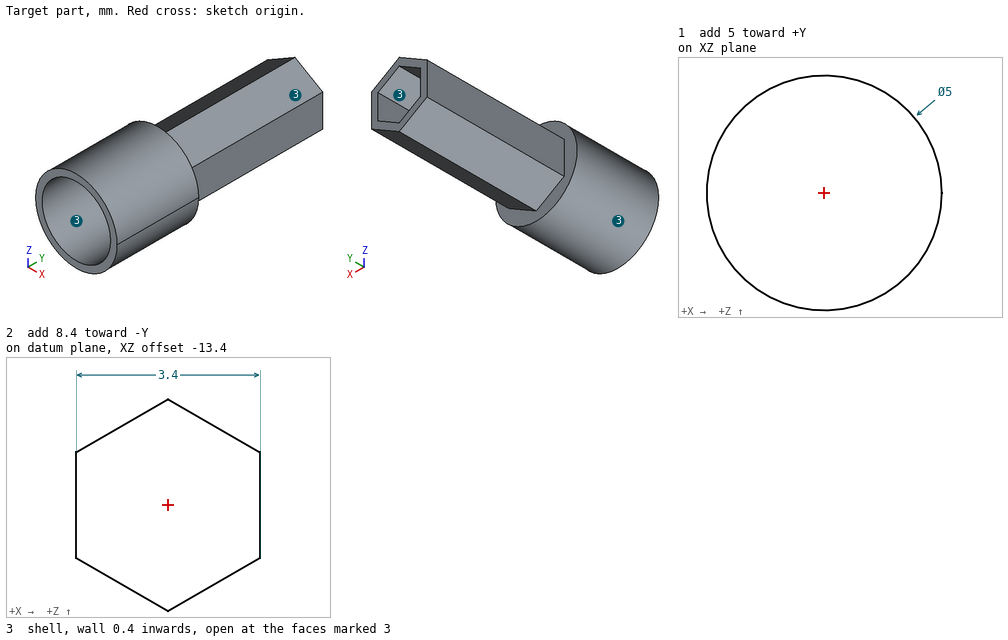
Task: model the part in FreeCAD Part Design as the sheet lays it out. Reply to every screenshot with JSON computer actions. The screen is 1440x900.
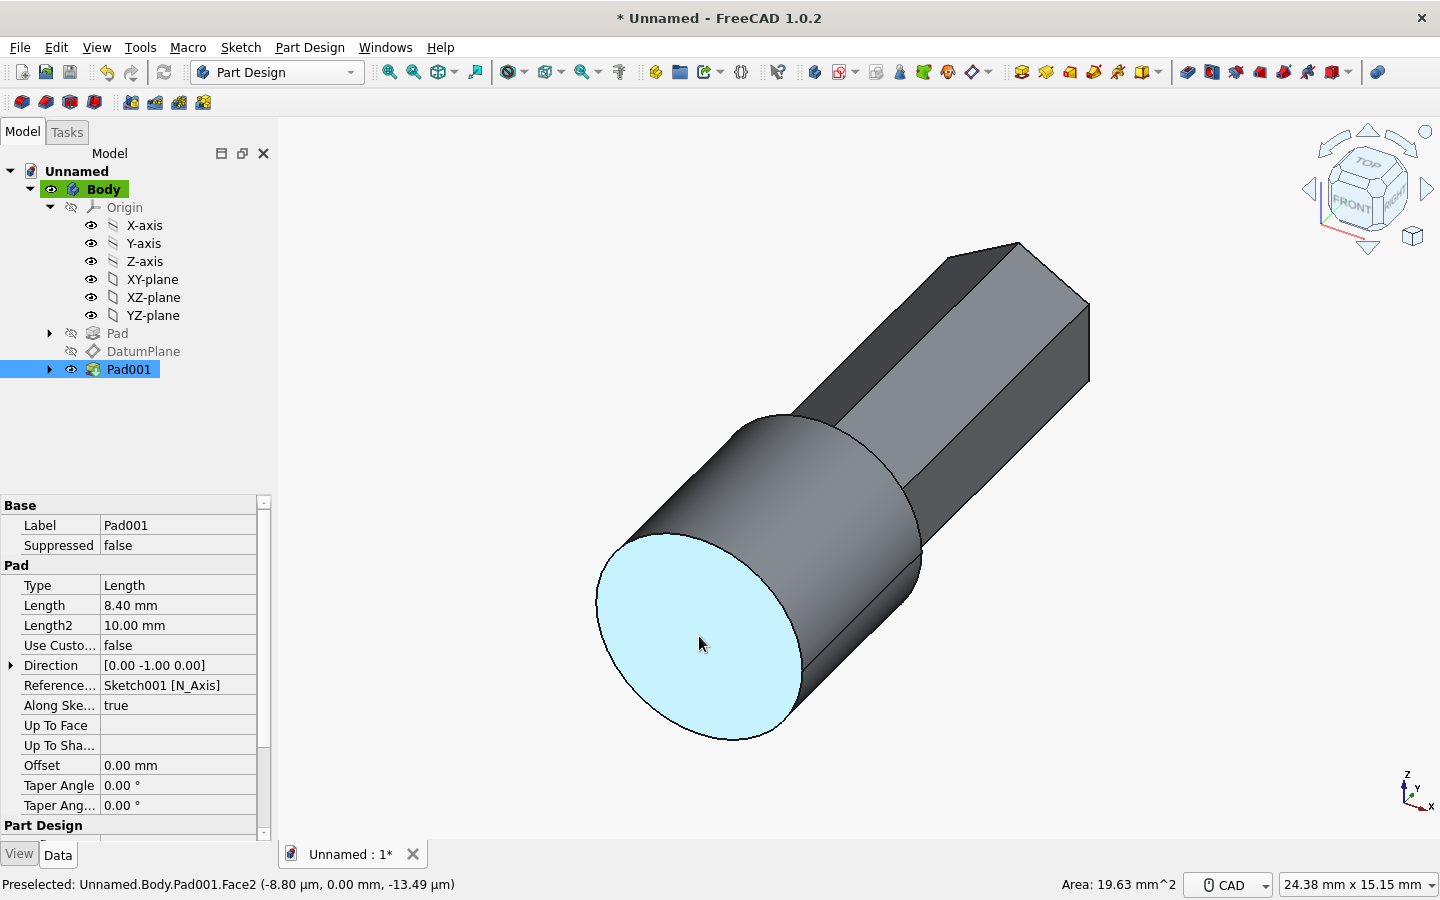
{"action": "key", "text": "0"}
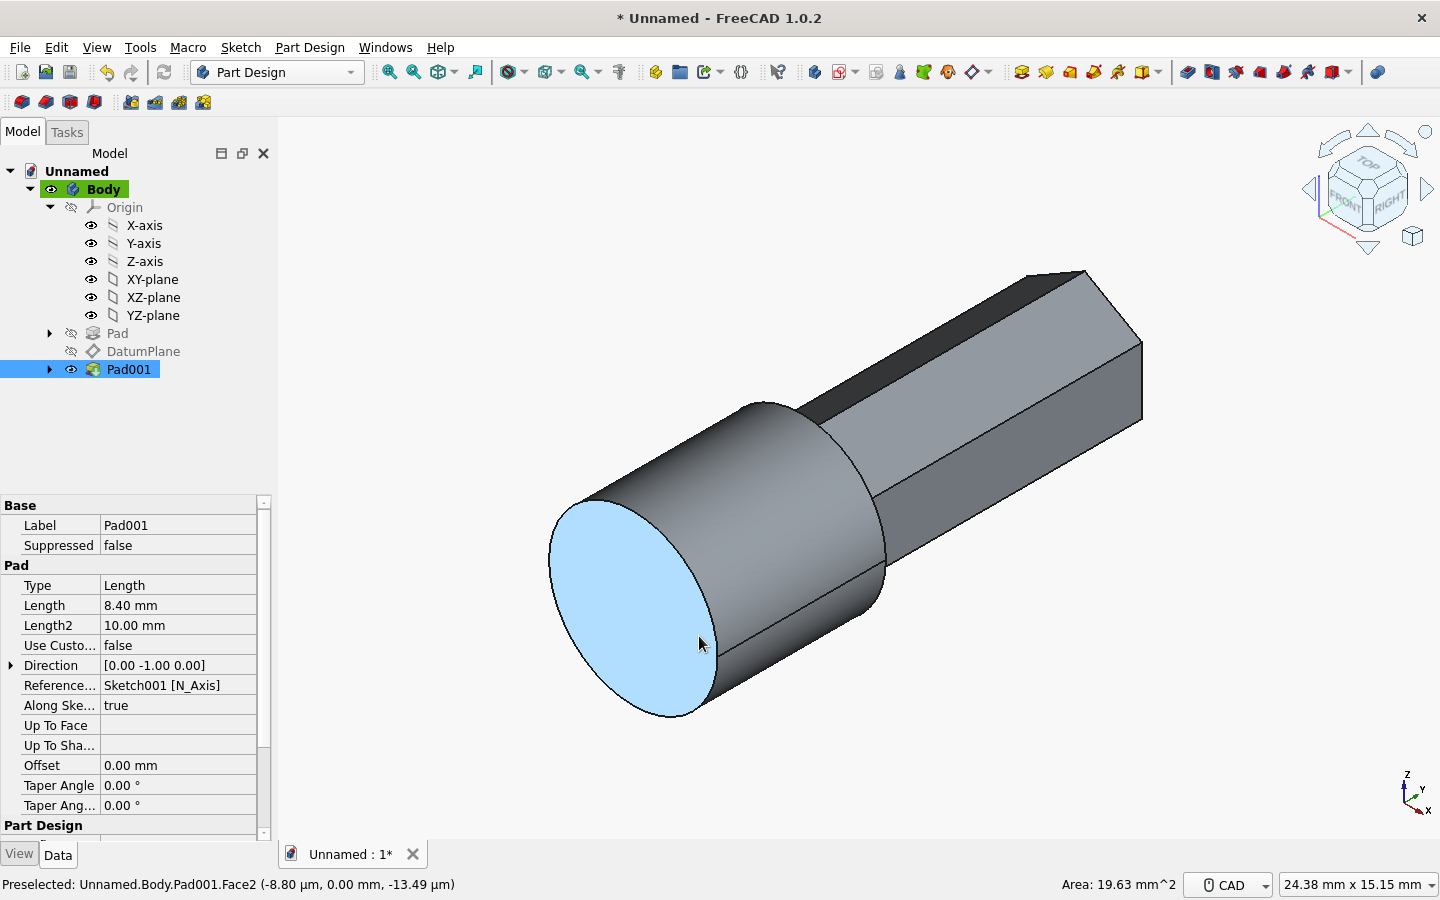
{"action": "key", "text": "2"}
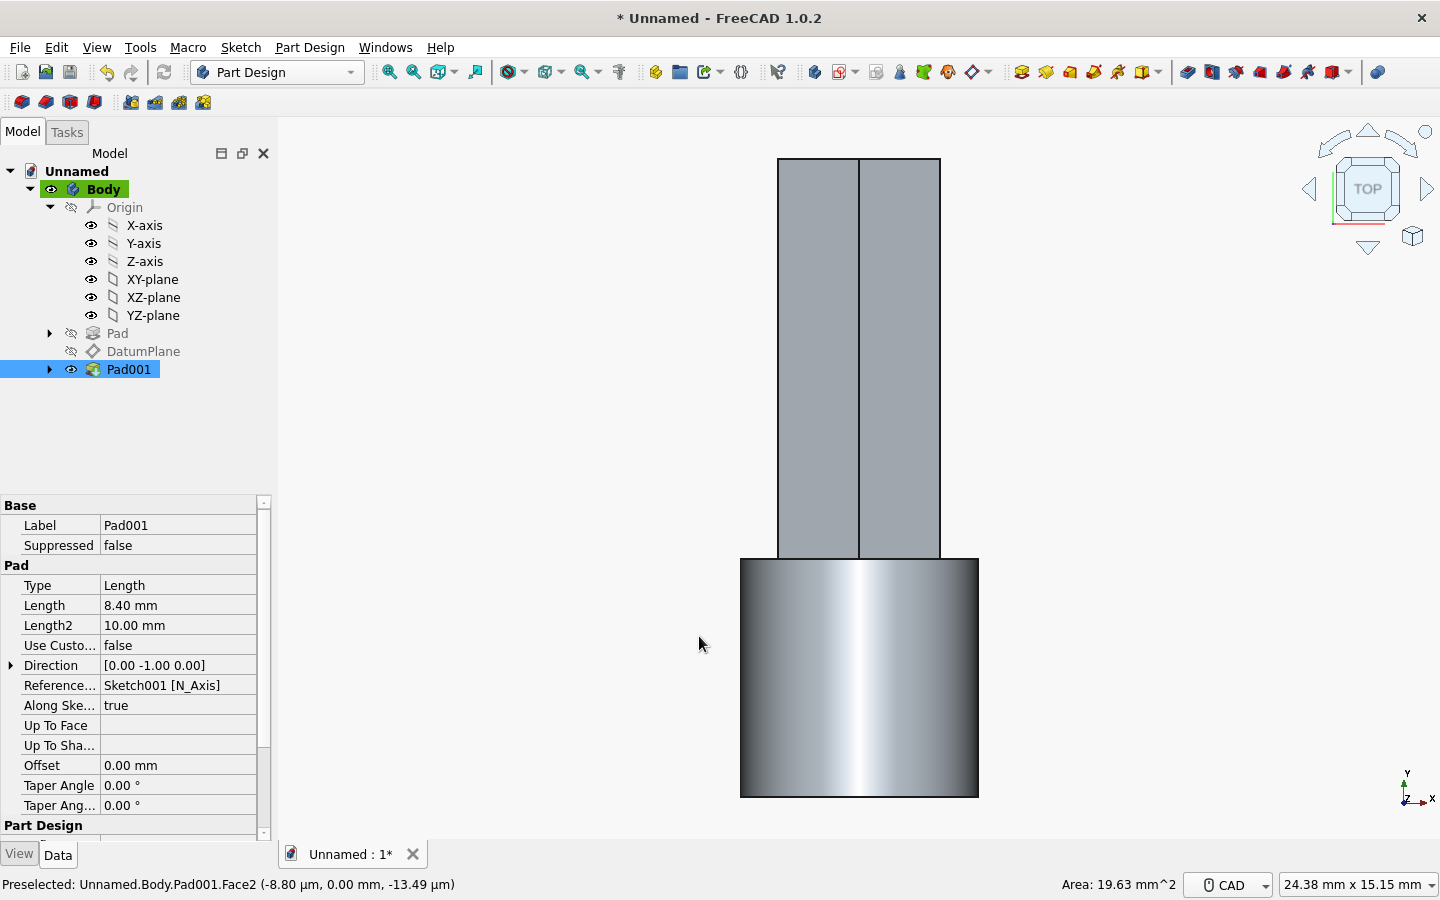
{"action": "key", "text": "1"}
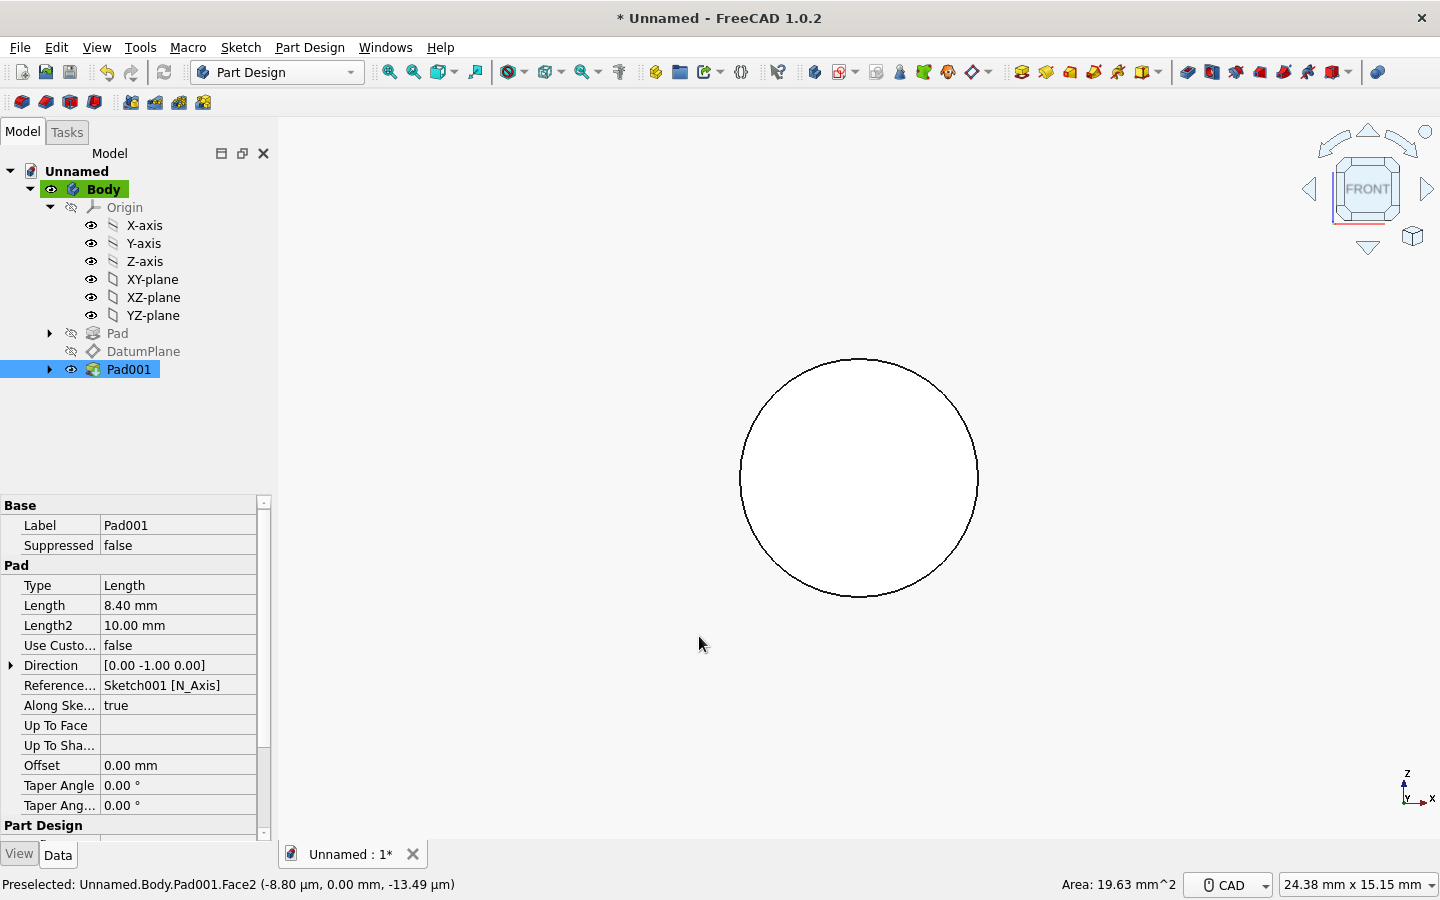
{"action": "left_click", "coordinate": [390, 72]}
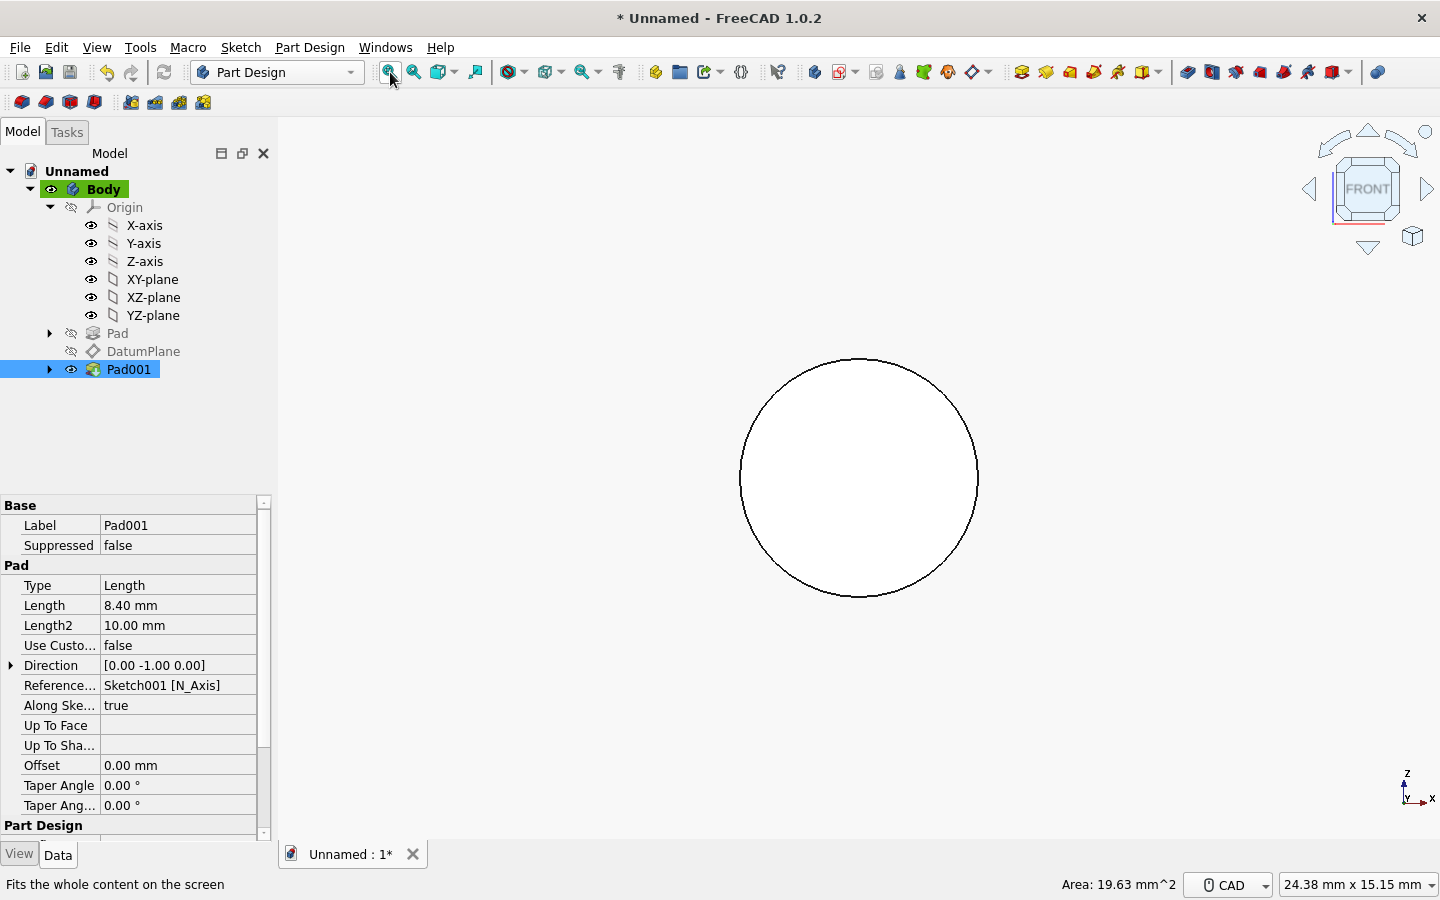
{"action": "key", "text": "3"}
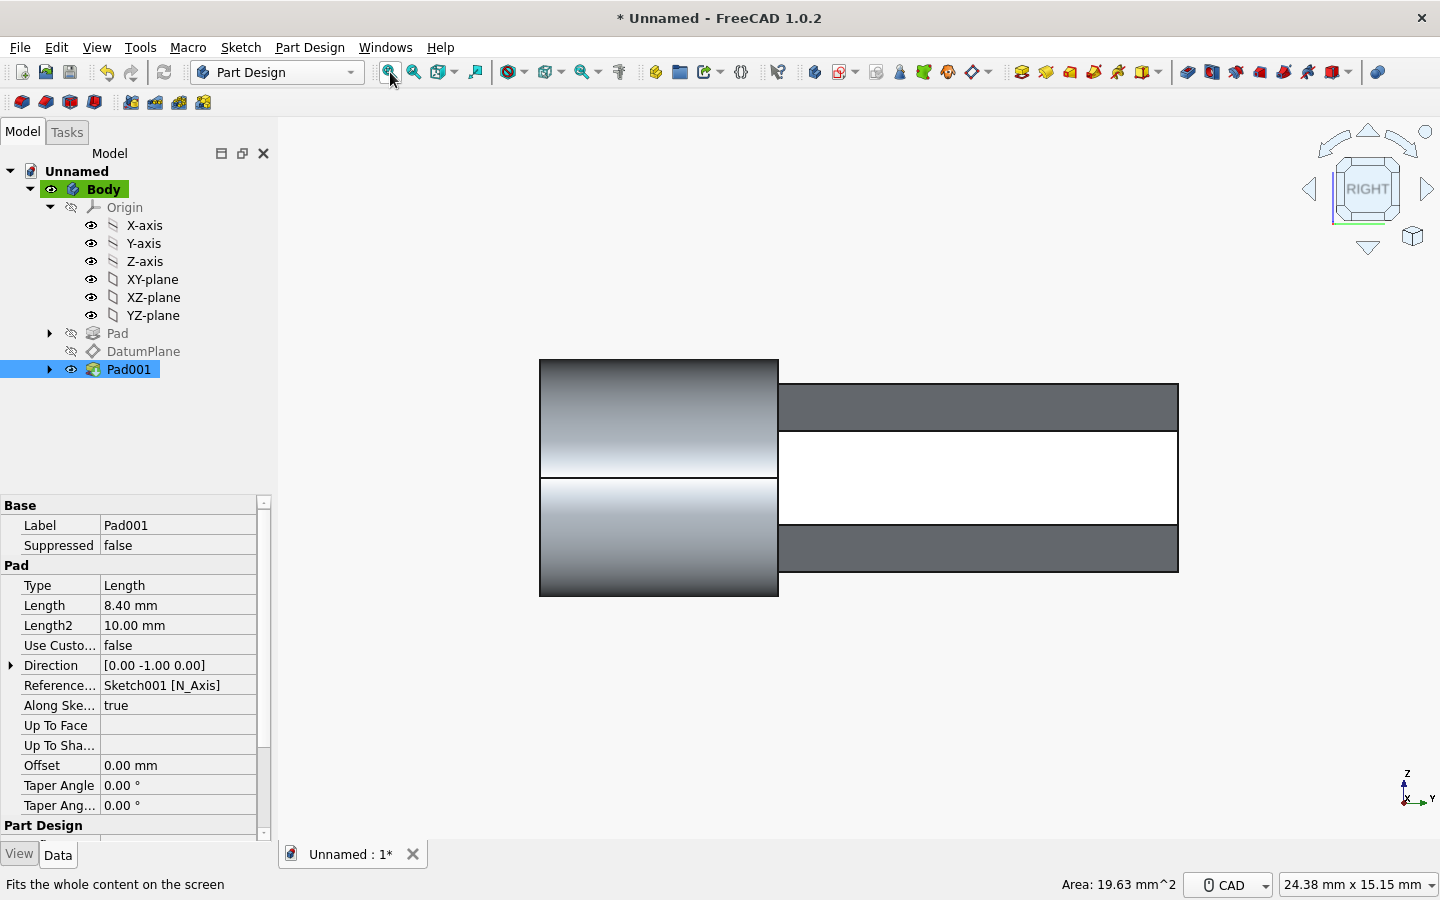
{"action": "key", "text": "5"}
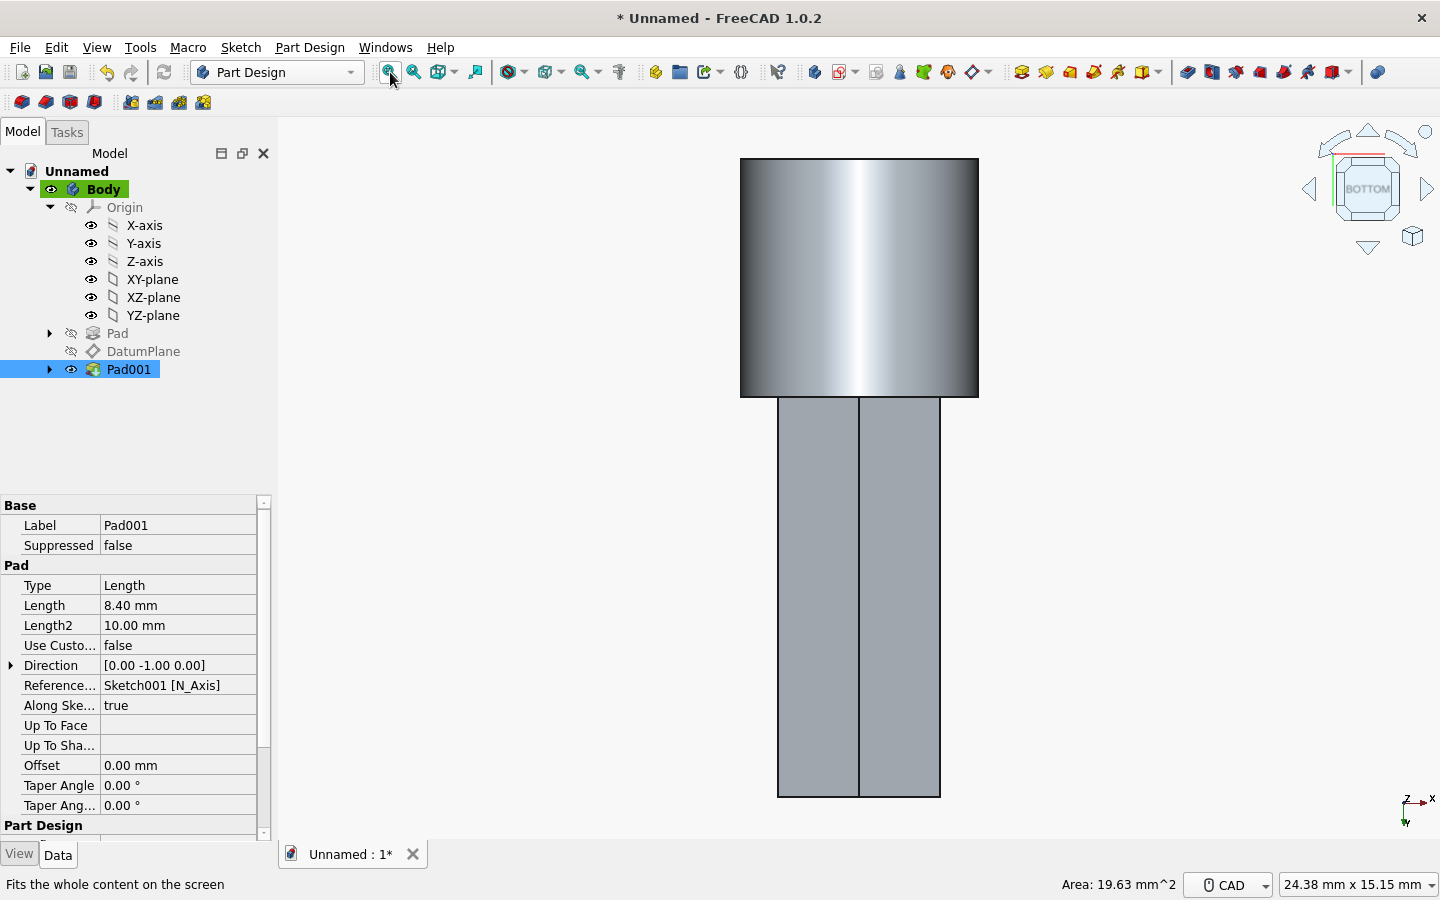
{"action": "key", "text": "4"}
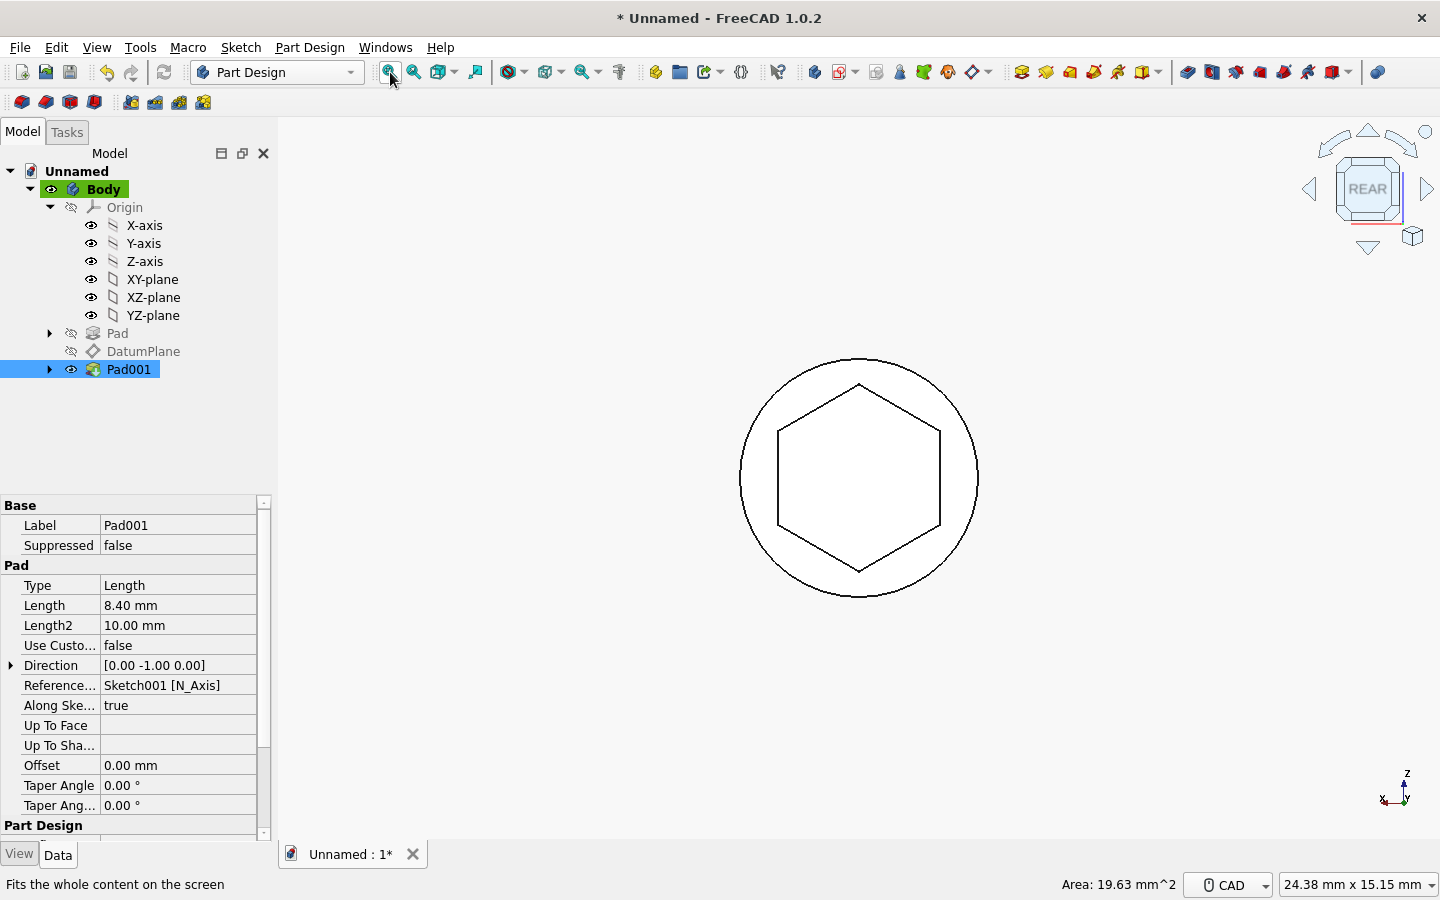
{"action": "left_click", "coordinate": [390, 72]}